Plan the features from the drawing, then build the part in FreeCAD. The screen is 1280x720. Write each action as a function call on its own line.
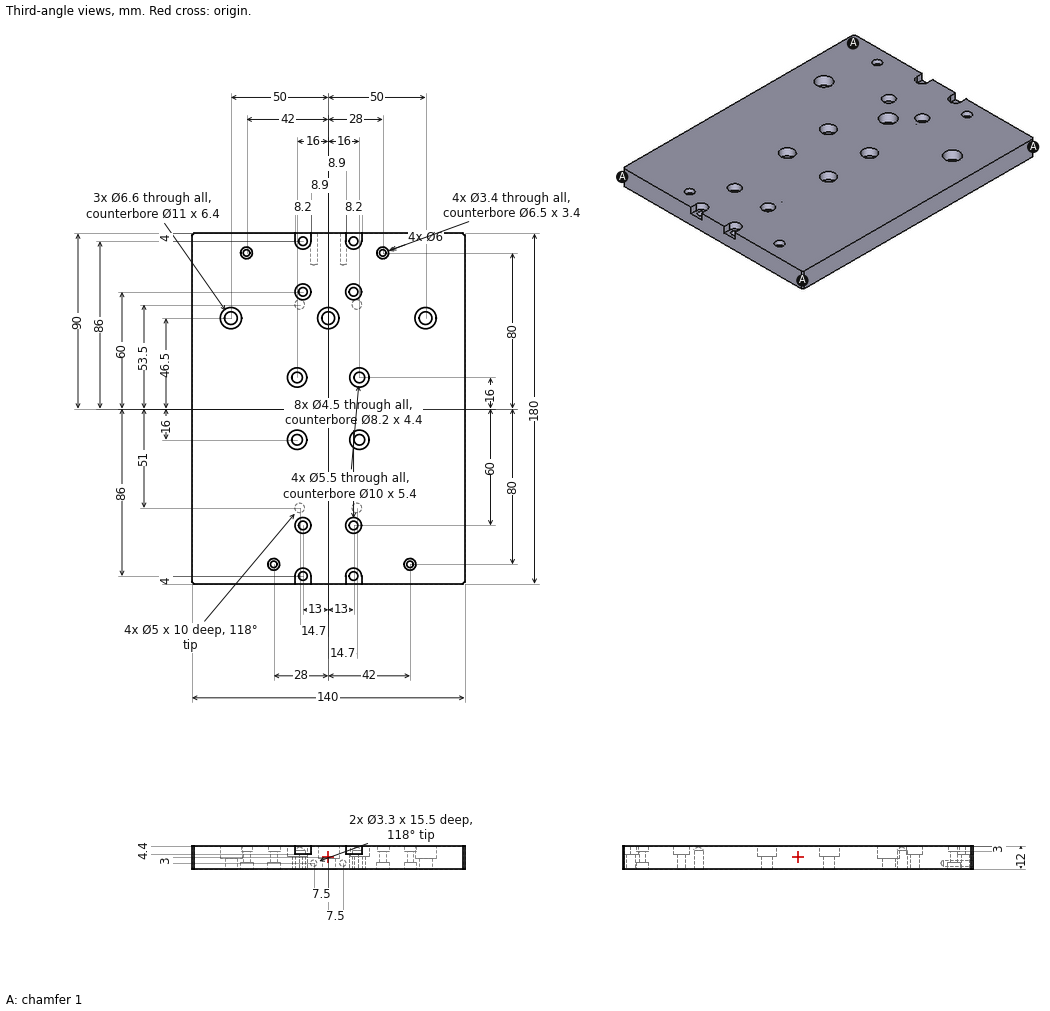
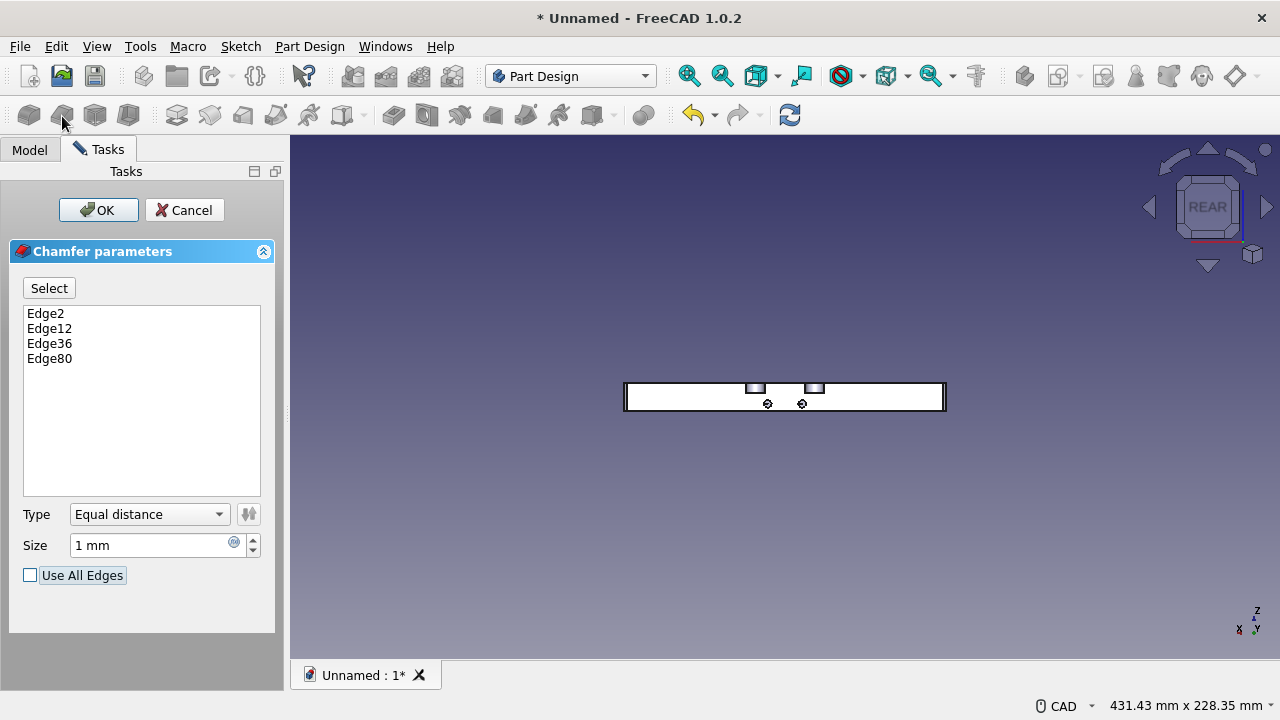
click(99, 210)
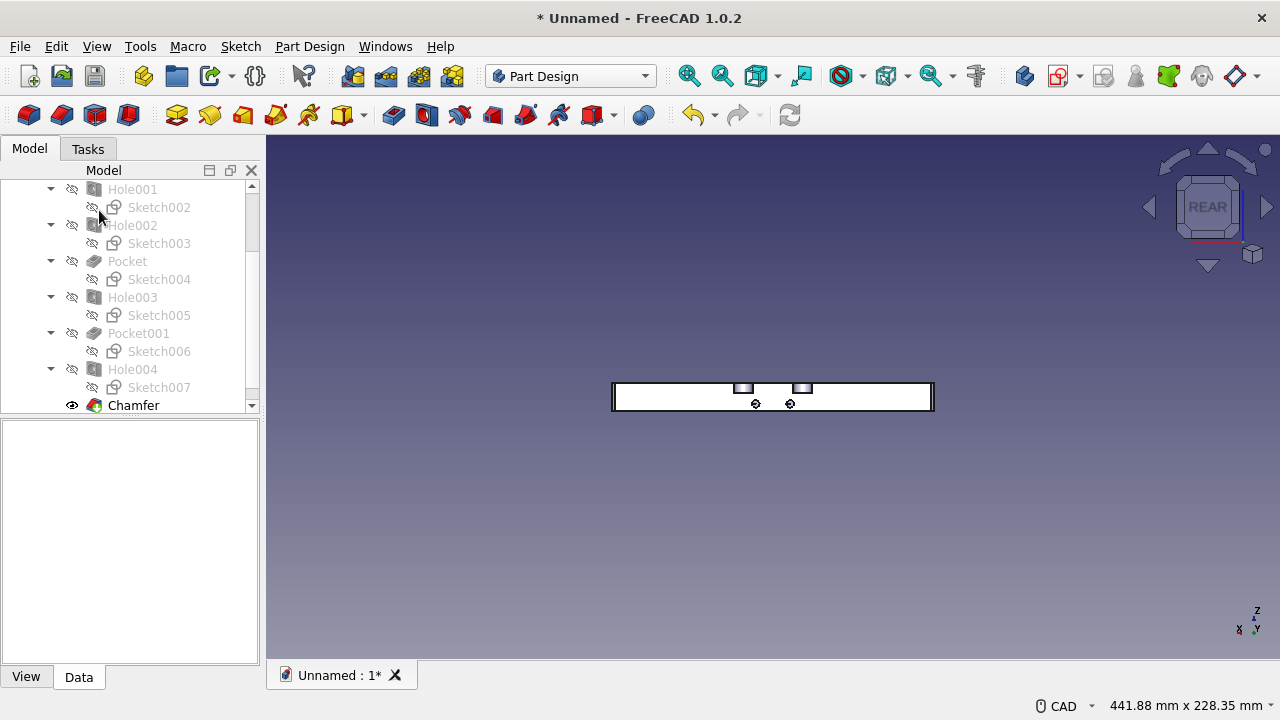
click(690, 76)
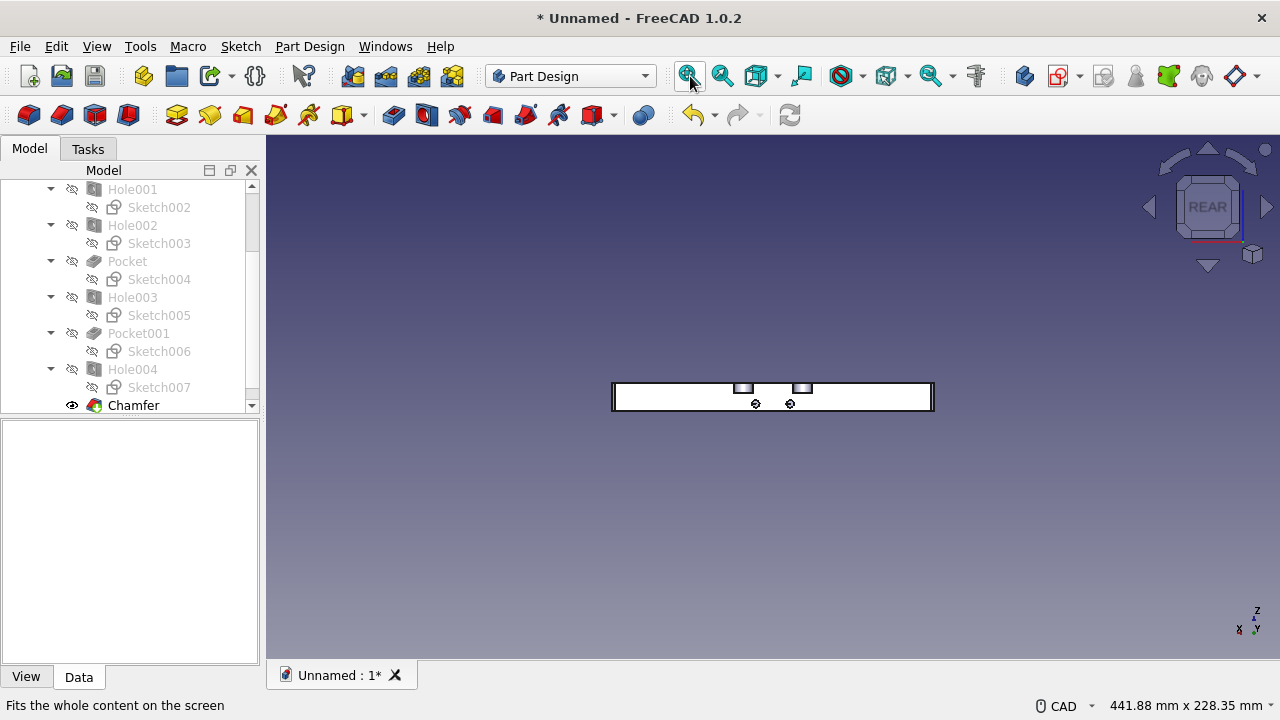
key(0)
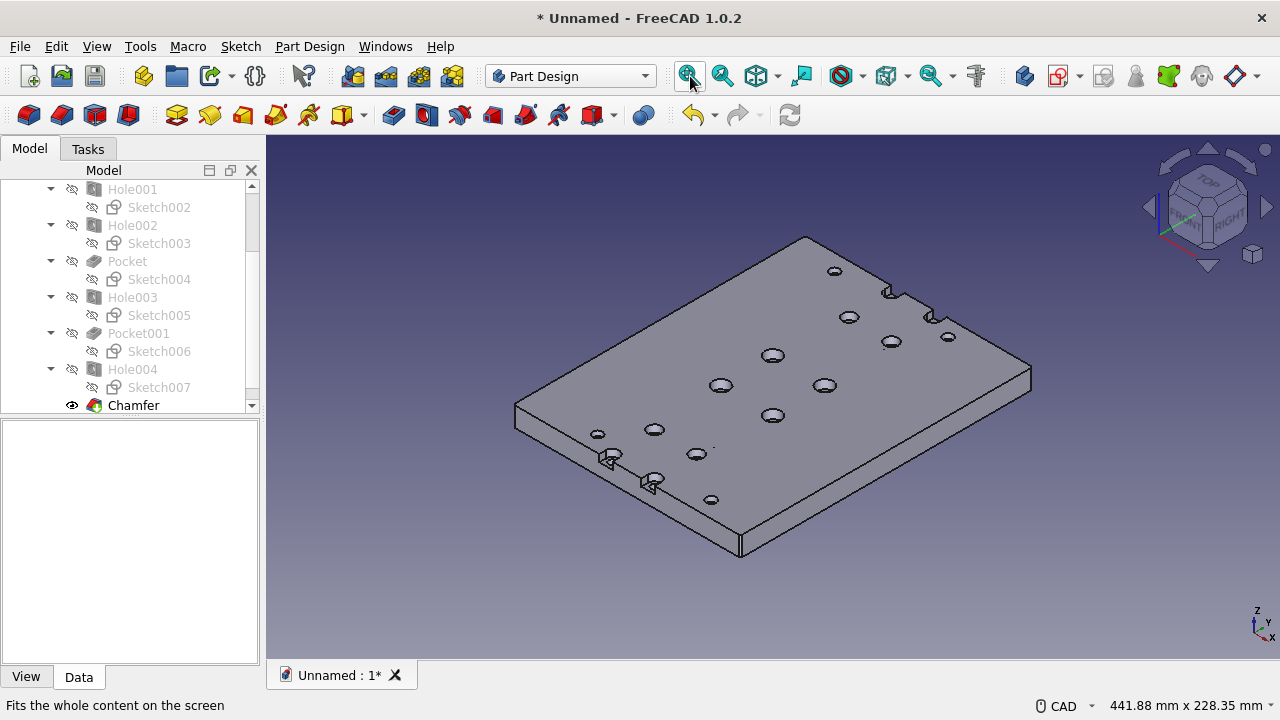
click(921, 374)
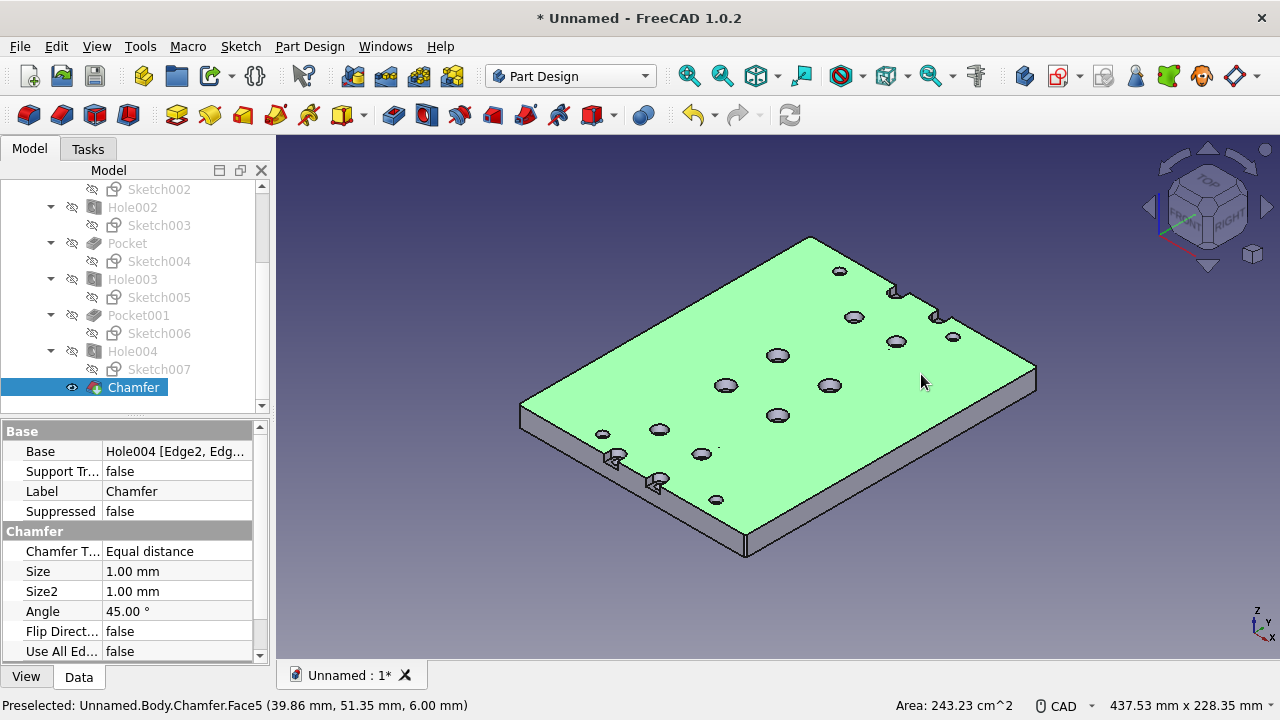
click(1058, 76)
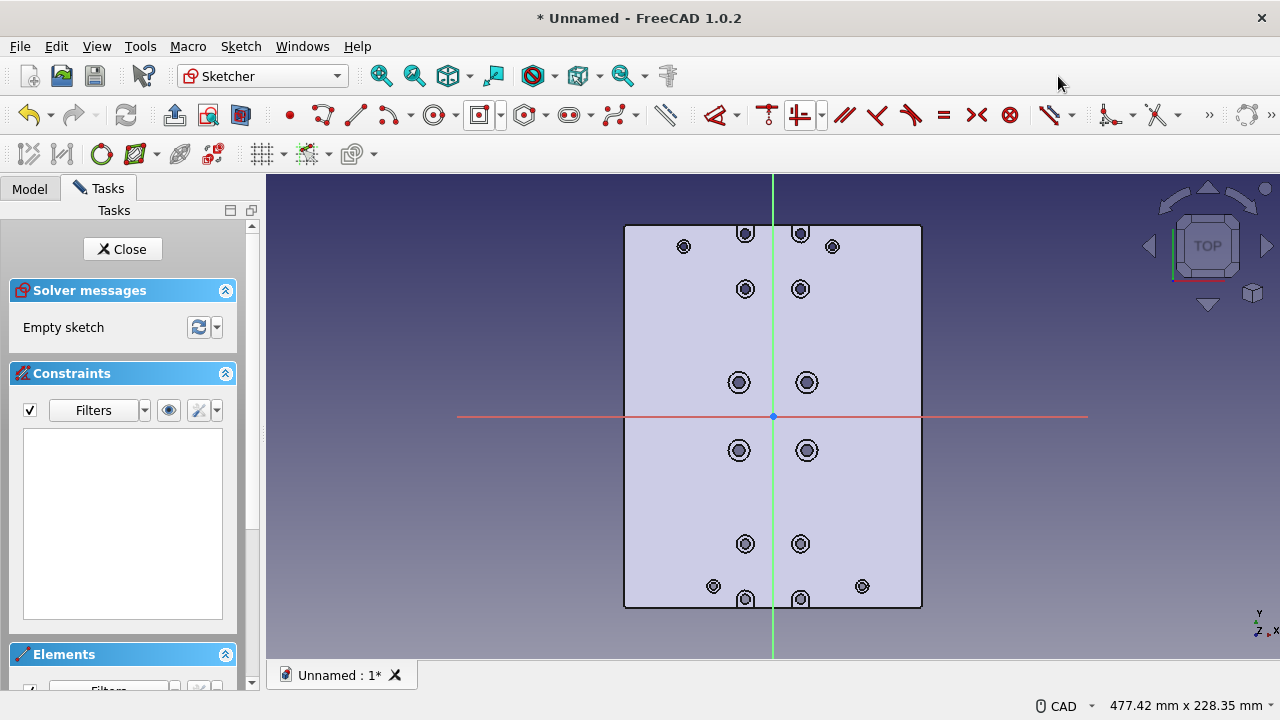
scroll(813, 333, up, 5)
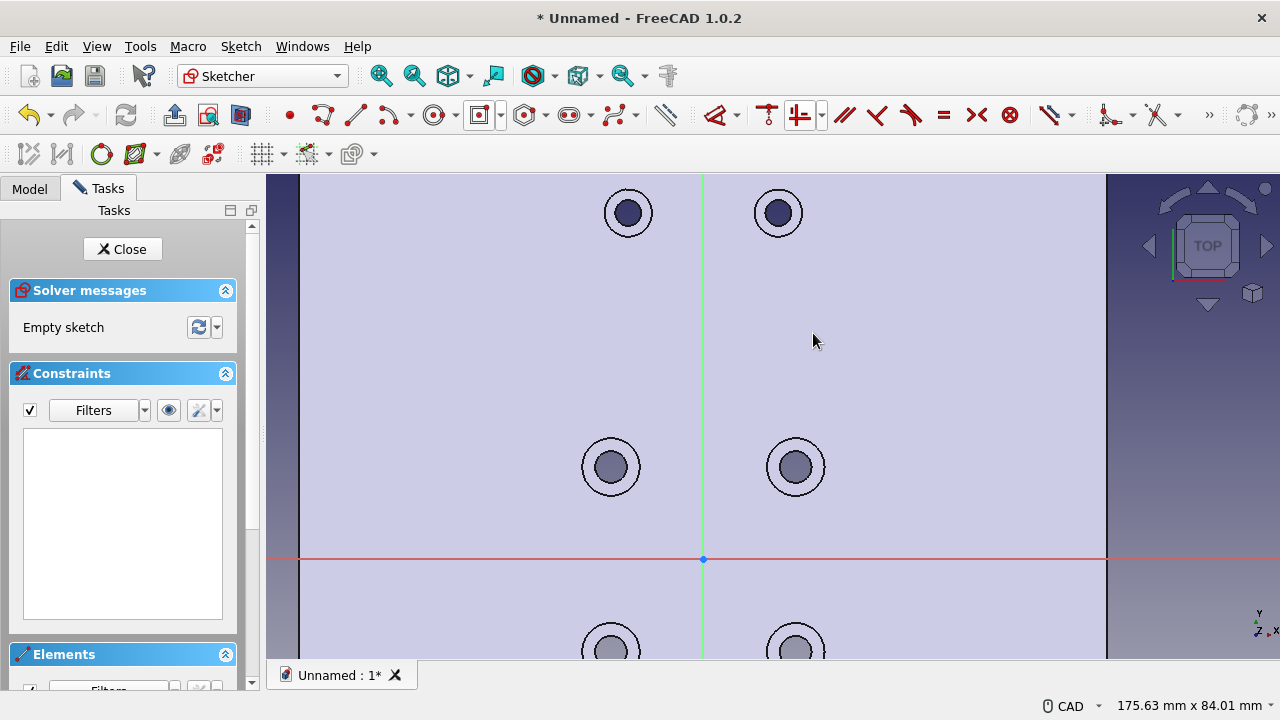
click(434, 116)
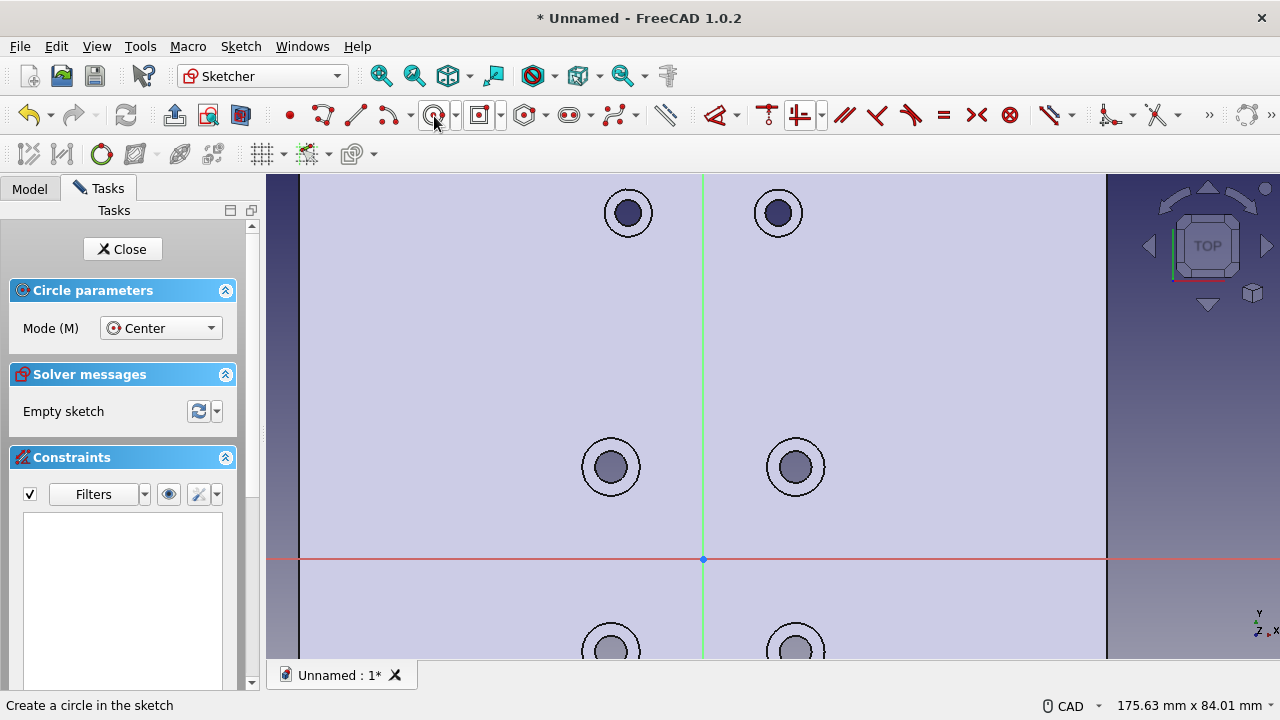
click(415, 291)
click(428, 277)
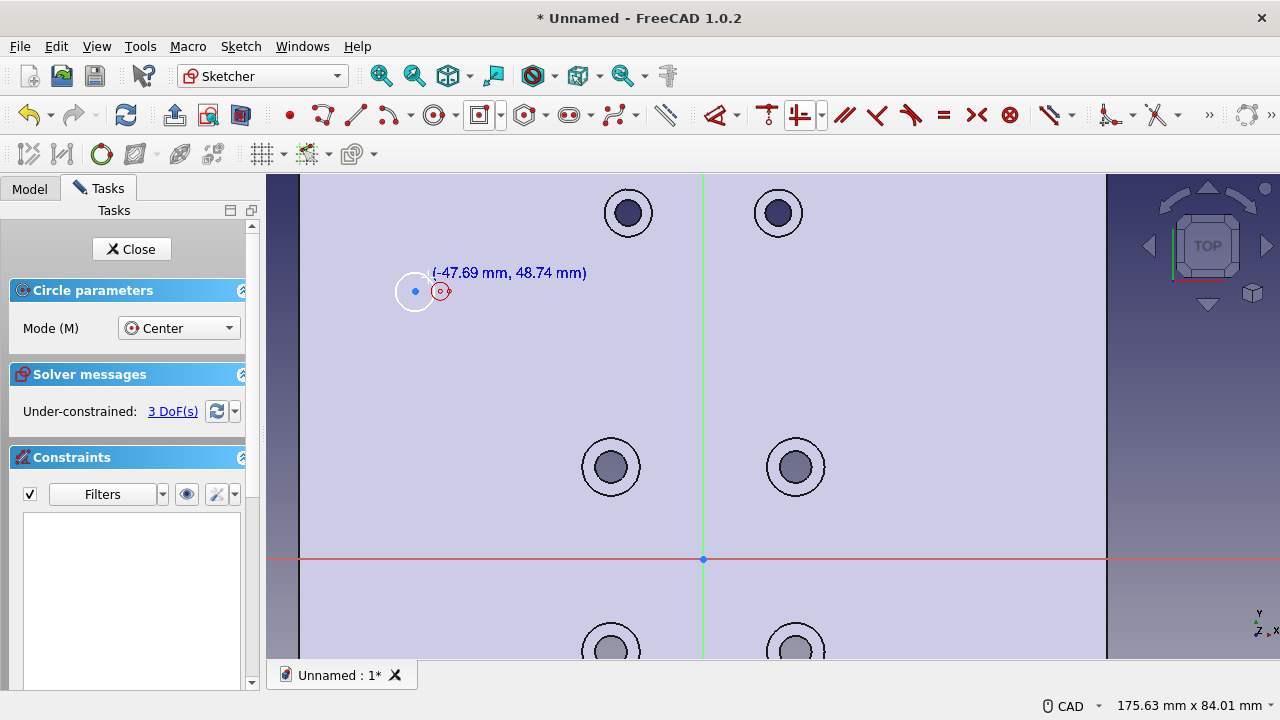
click(703, 291)
click(721, 284)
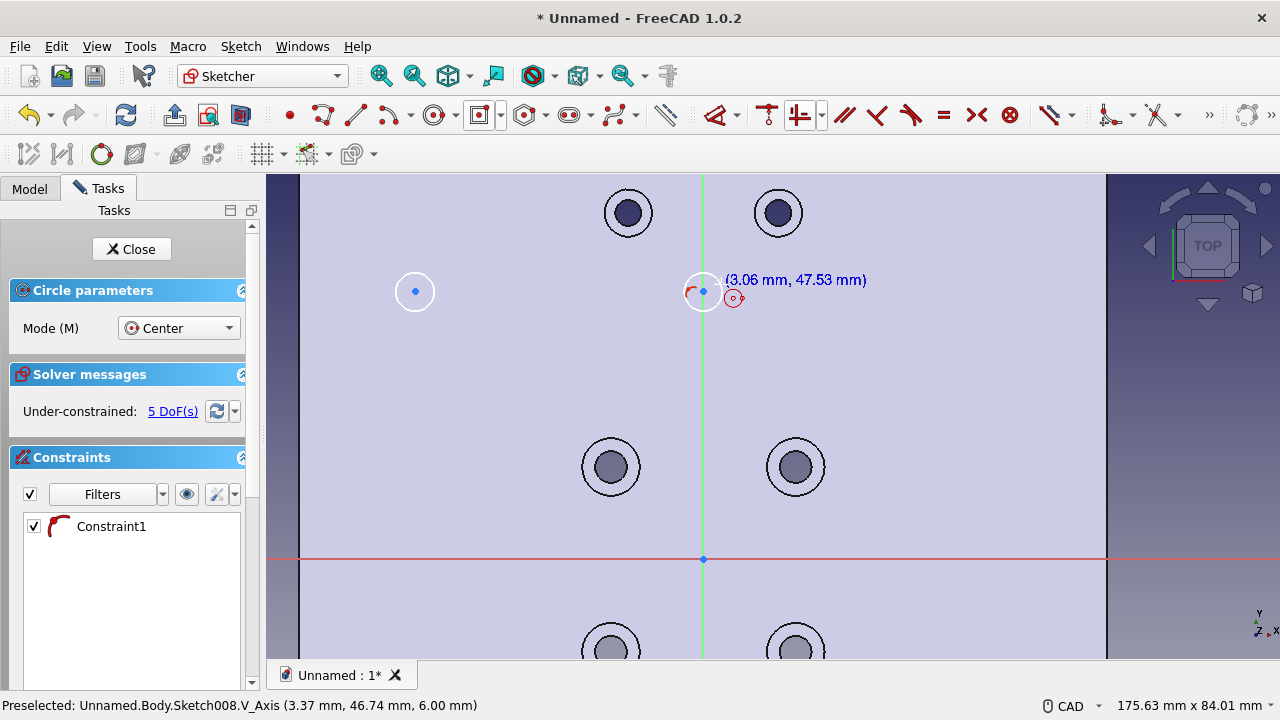
click(992, 291)
click(1005, 277)
key(Escape)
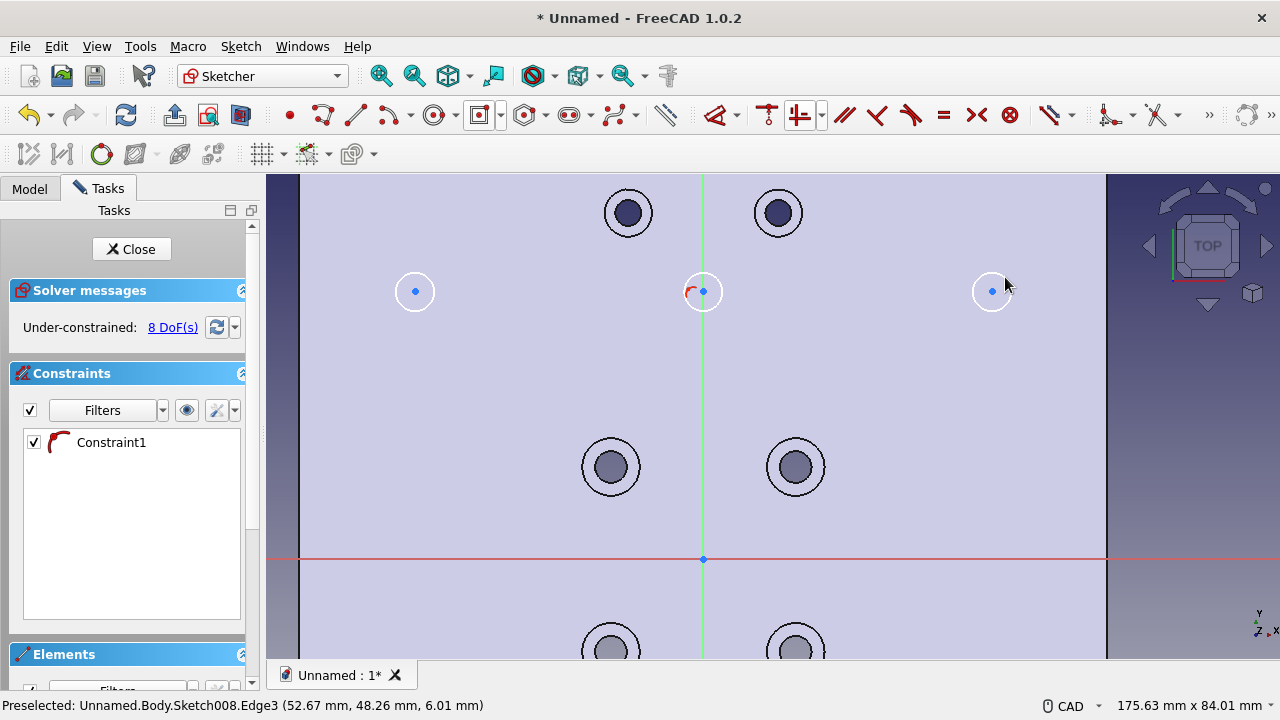
click(428, 278)